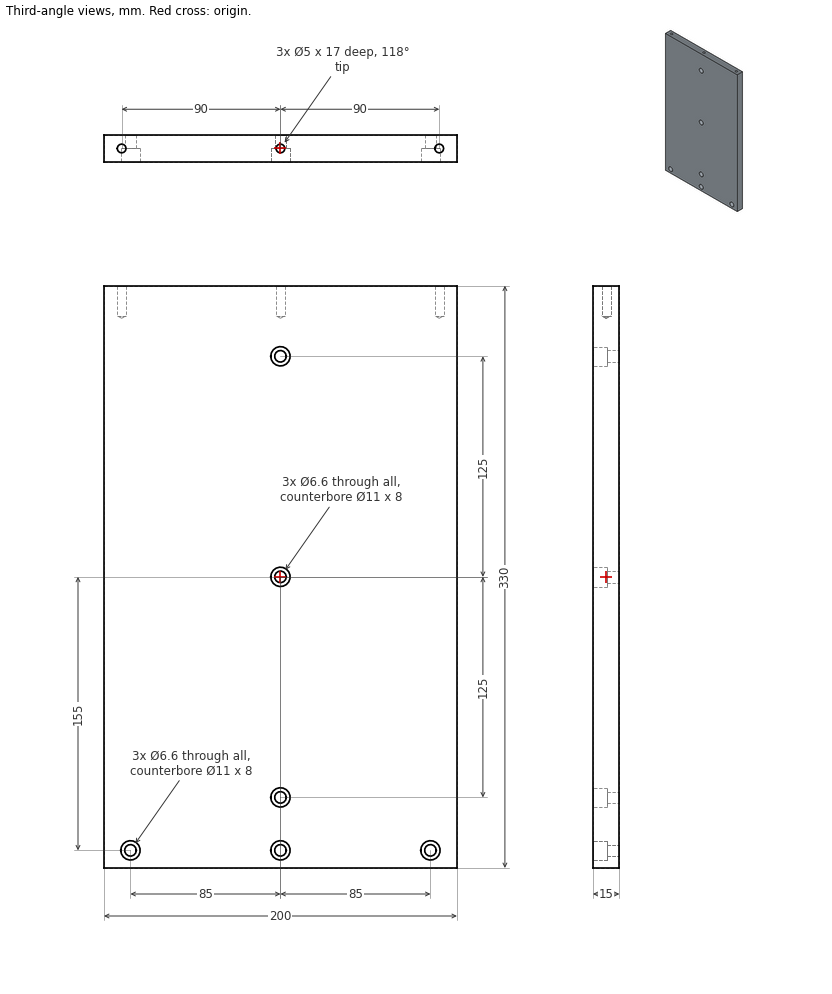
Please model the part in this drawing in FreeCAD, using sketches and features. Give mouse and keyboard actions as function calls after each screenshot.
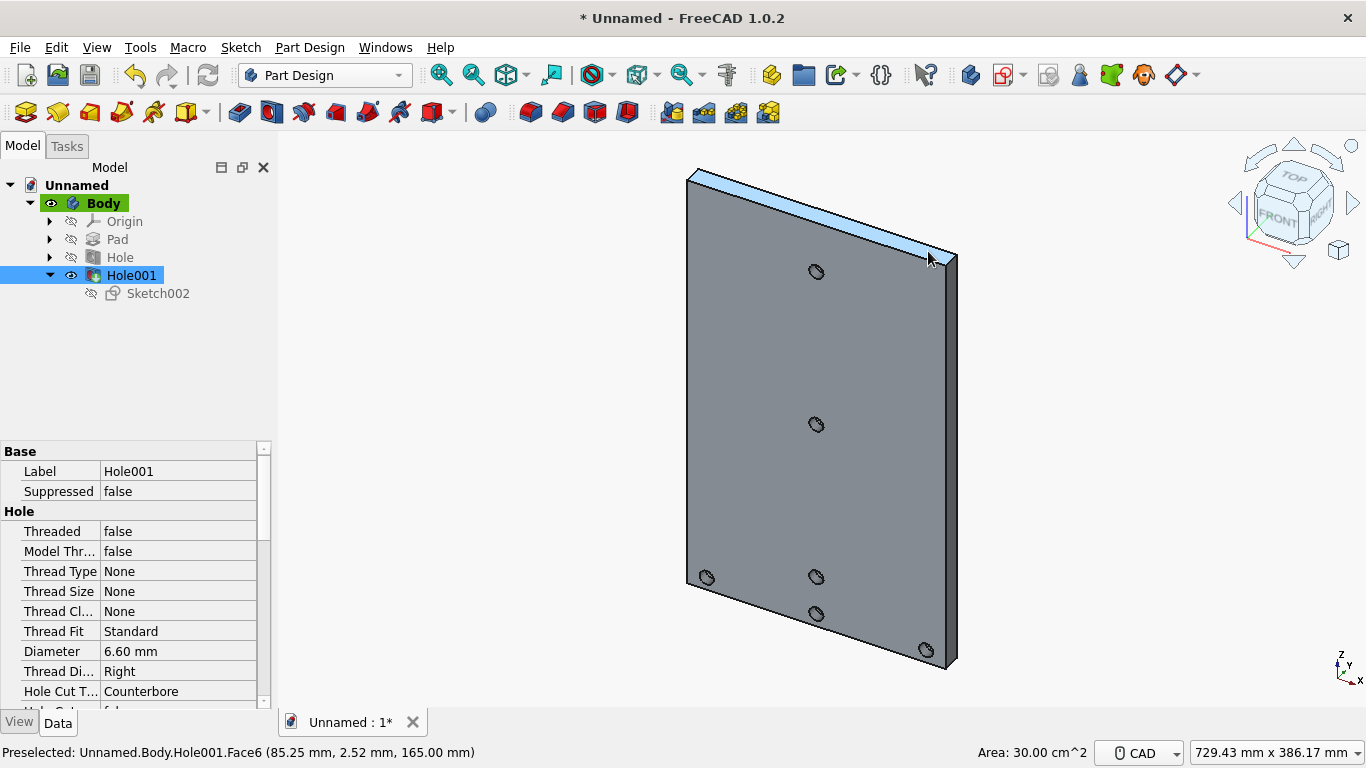
click(1004, 76)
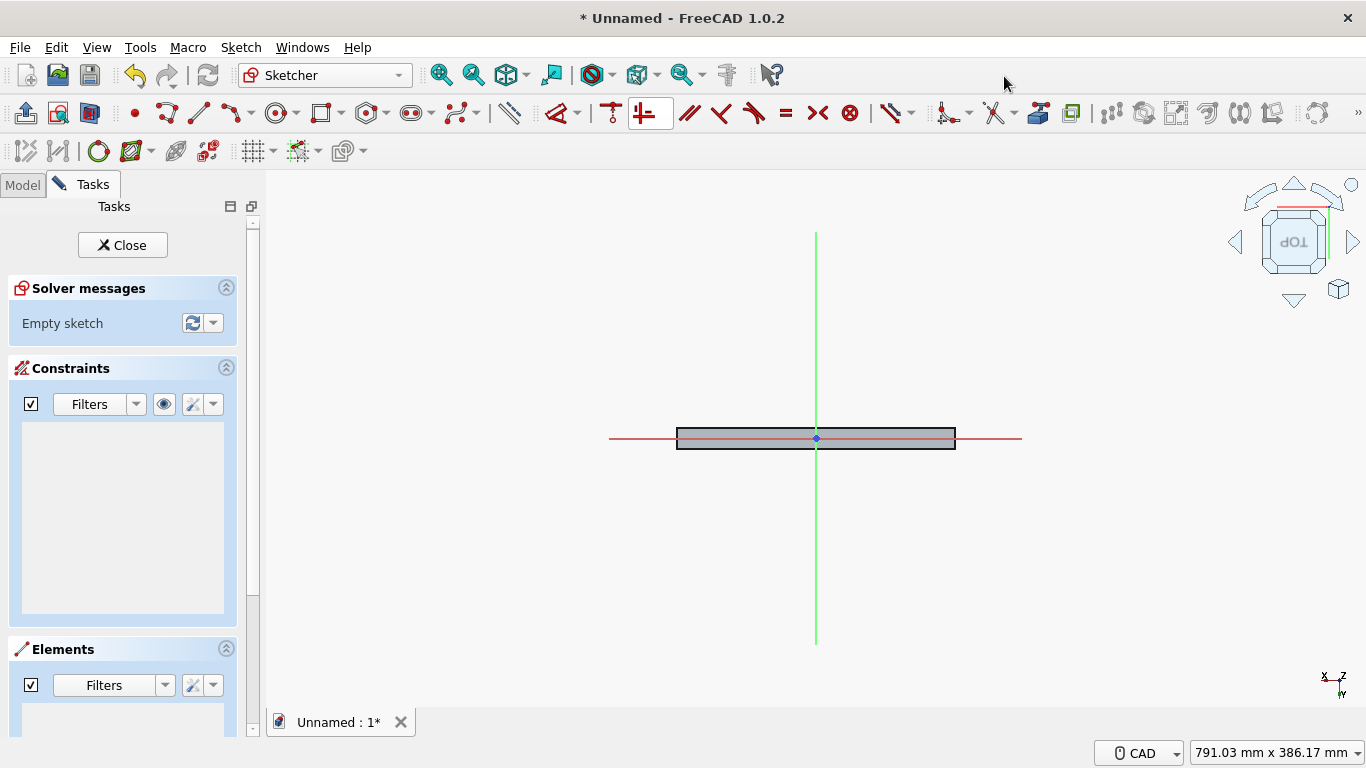
scroll(856, 439, up, 5)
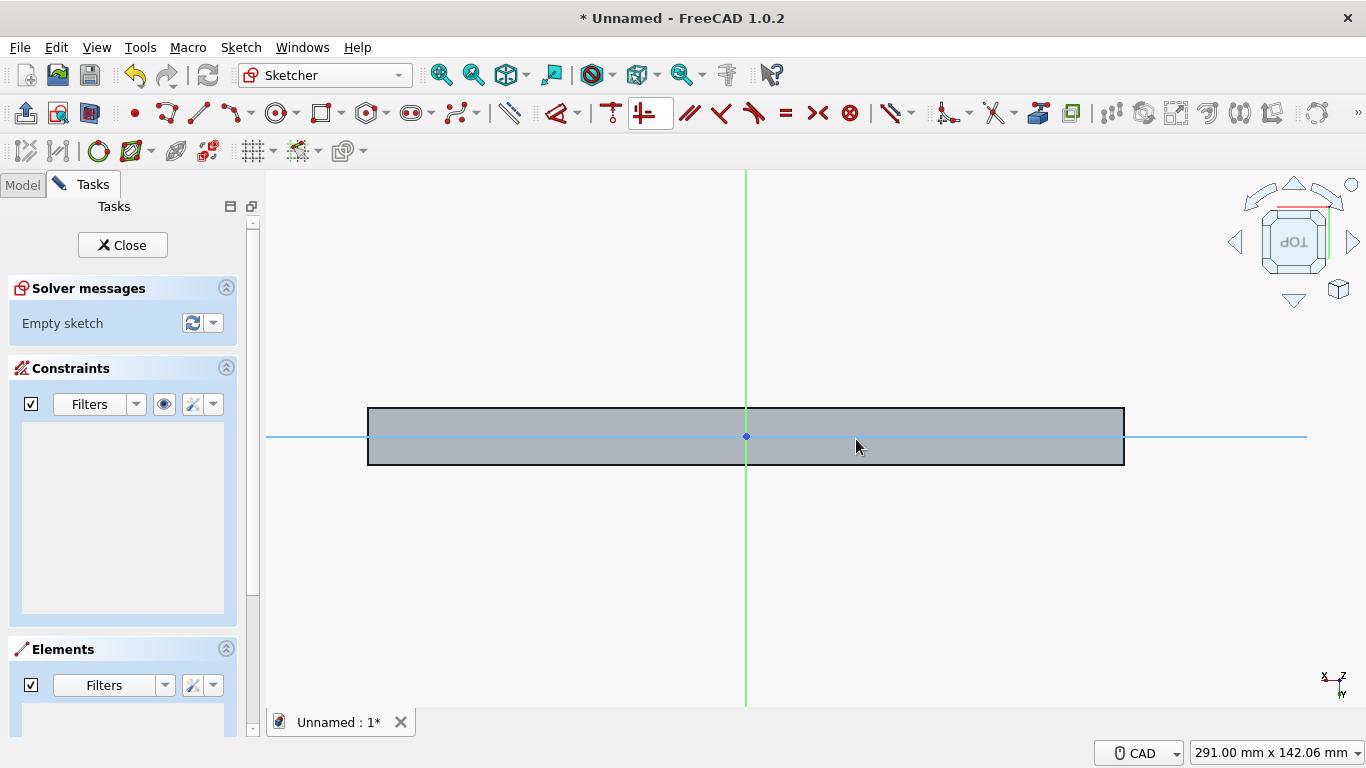
key(g)
key(c)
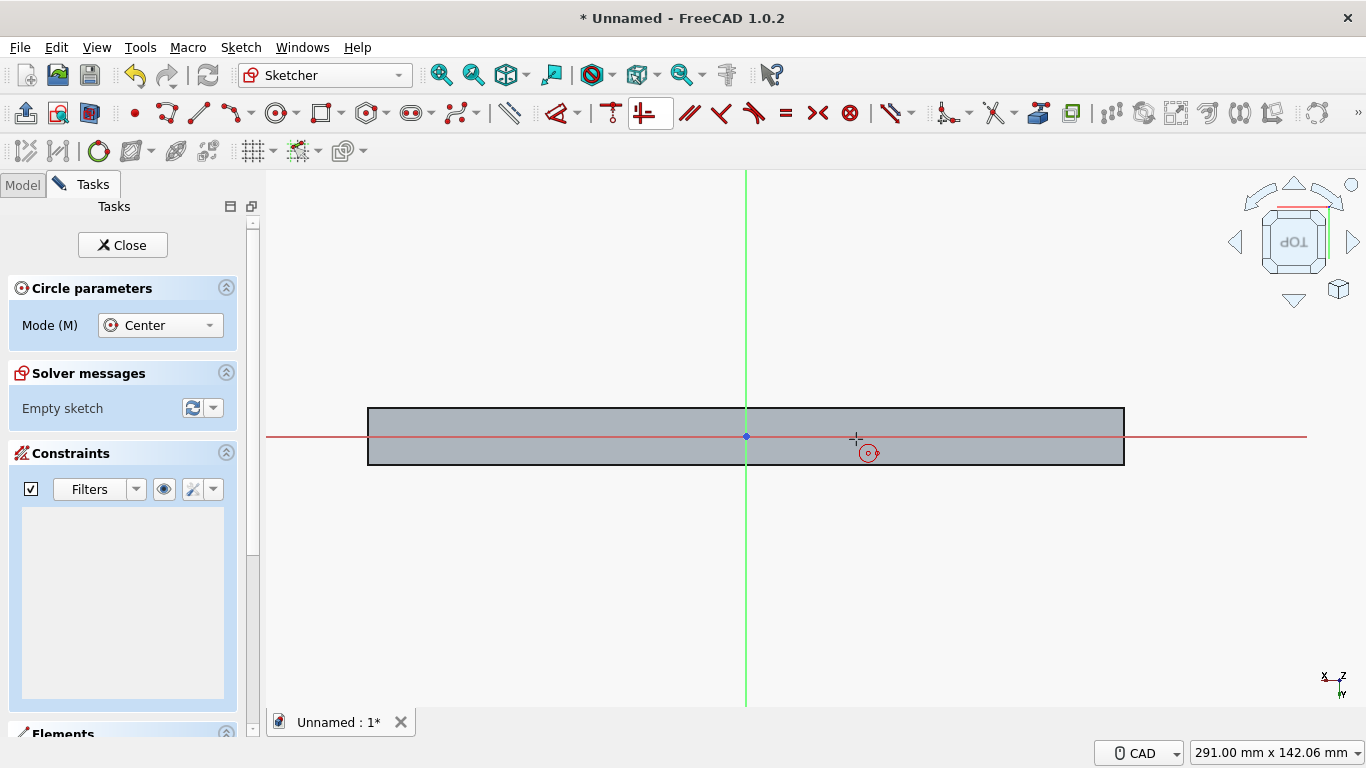
scroll(746, 437, up, 5)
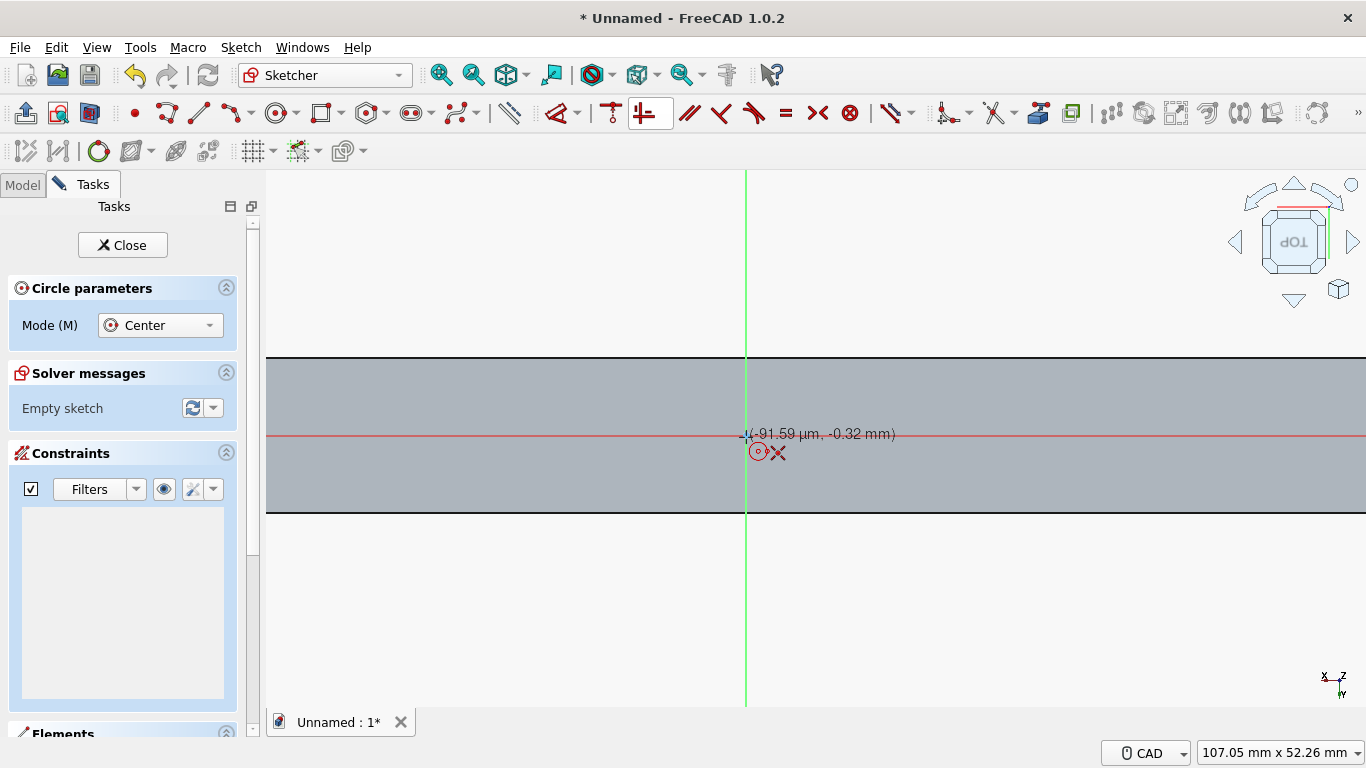
click(746, 436)
click(764, 417)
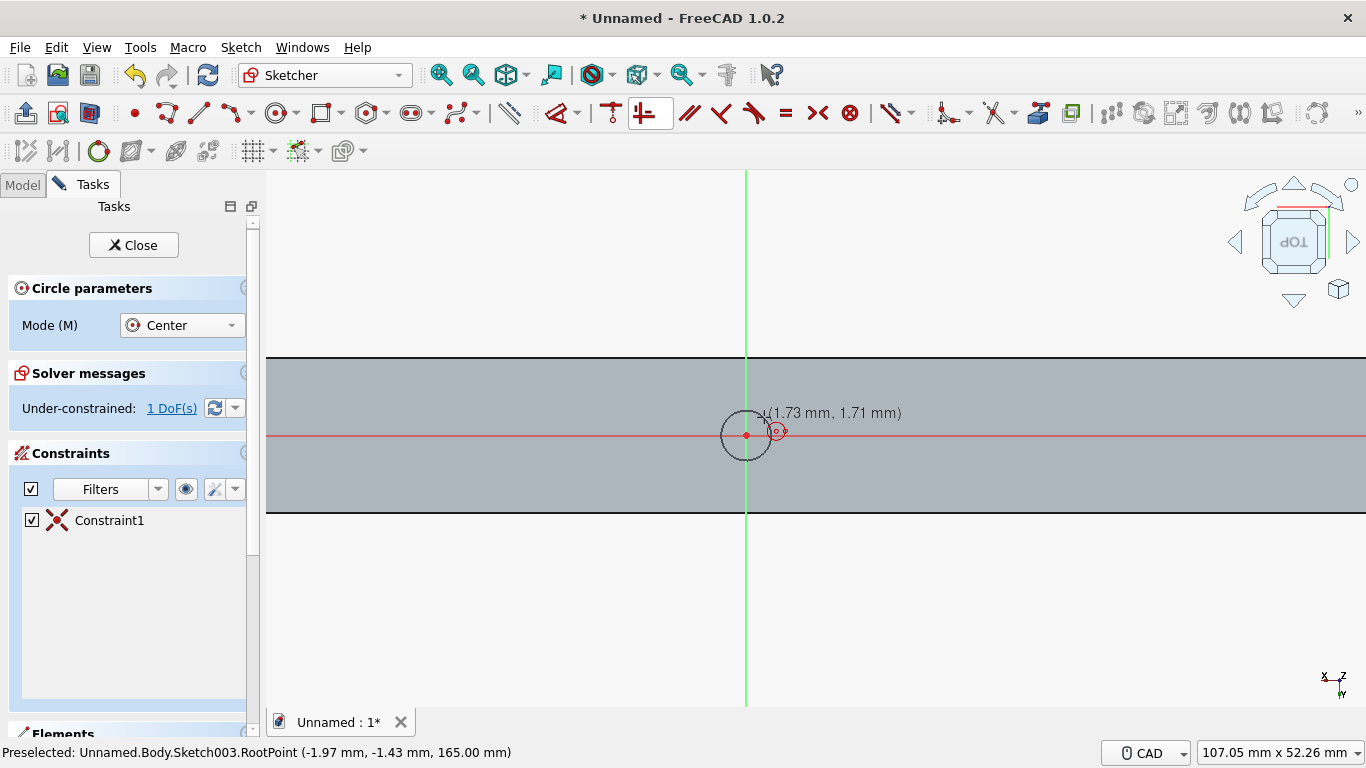
scroll(748, 440, down, 5)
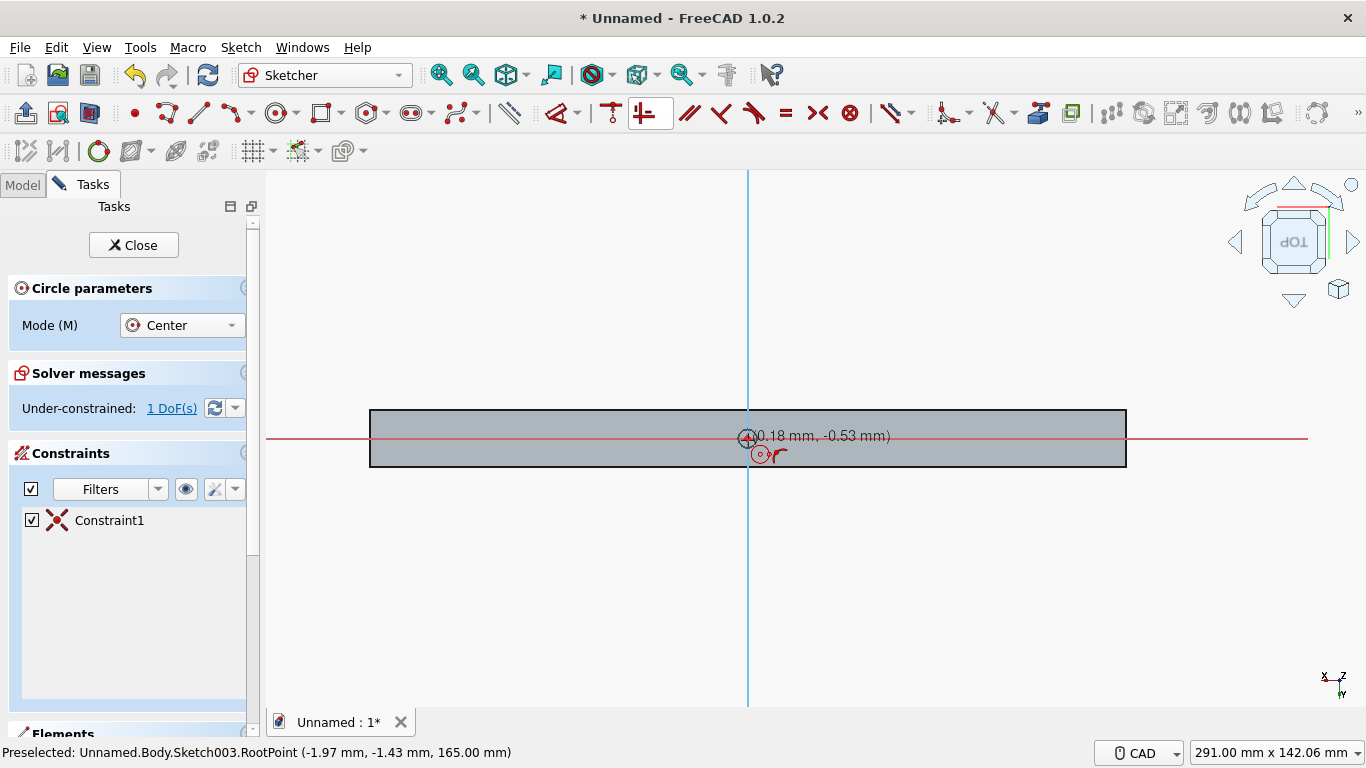
scroll(1088, 439, up, 5)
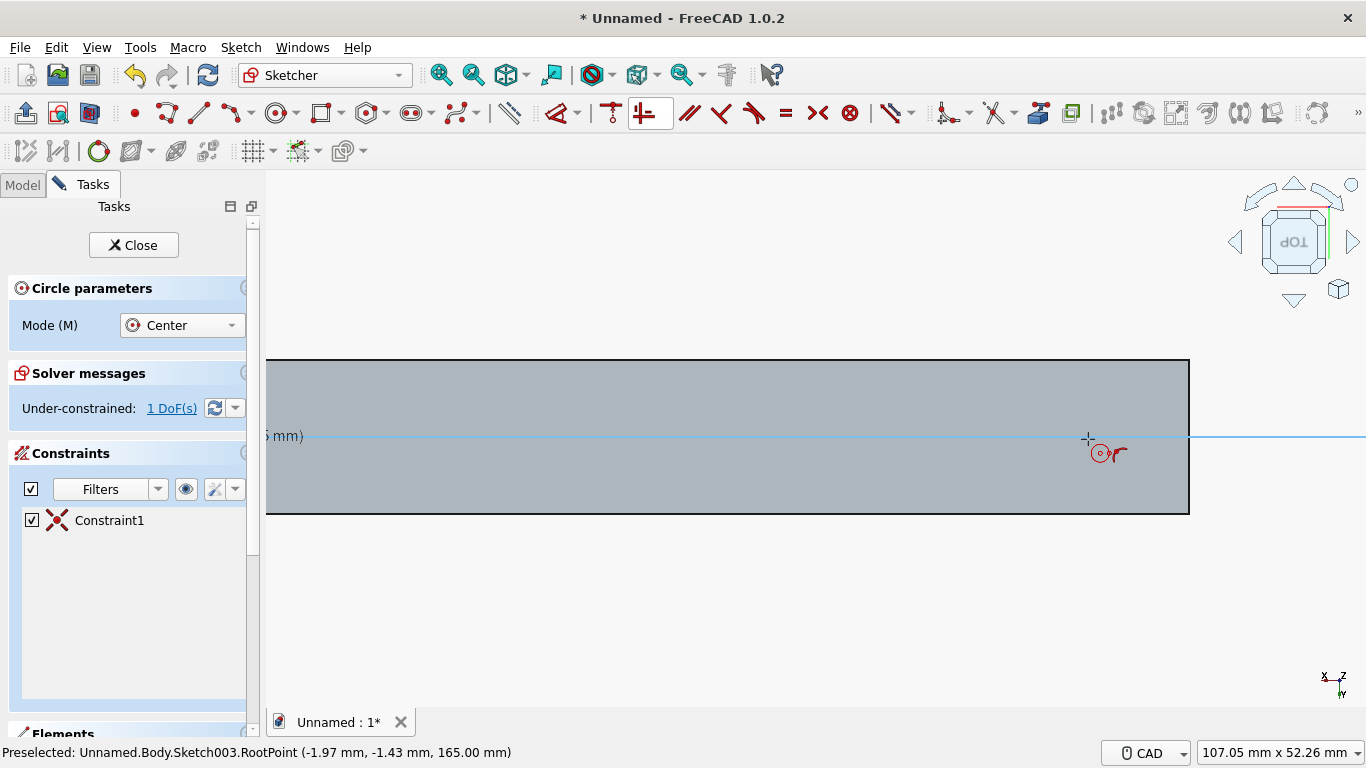
click(1086, 437)
click(1104, 419)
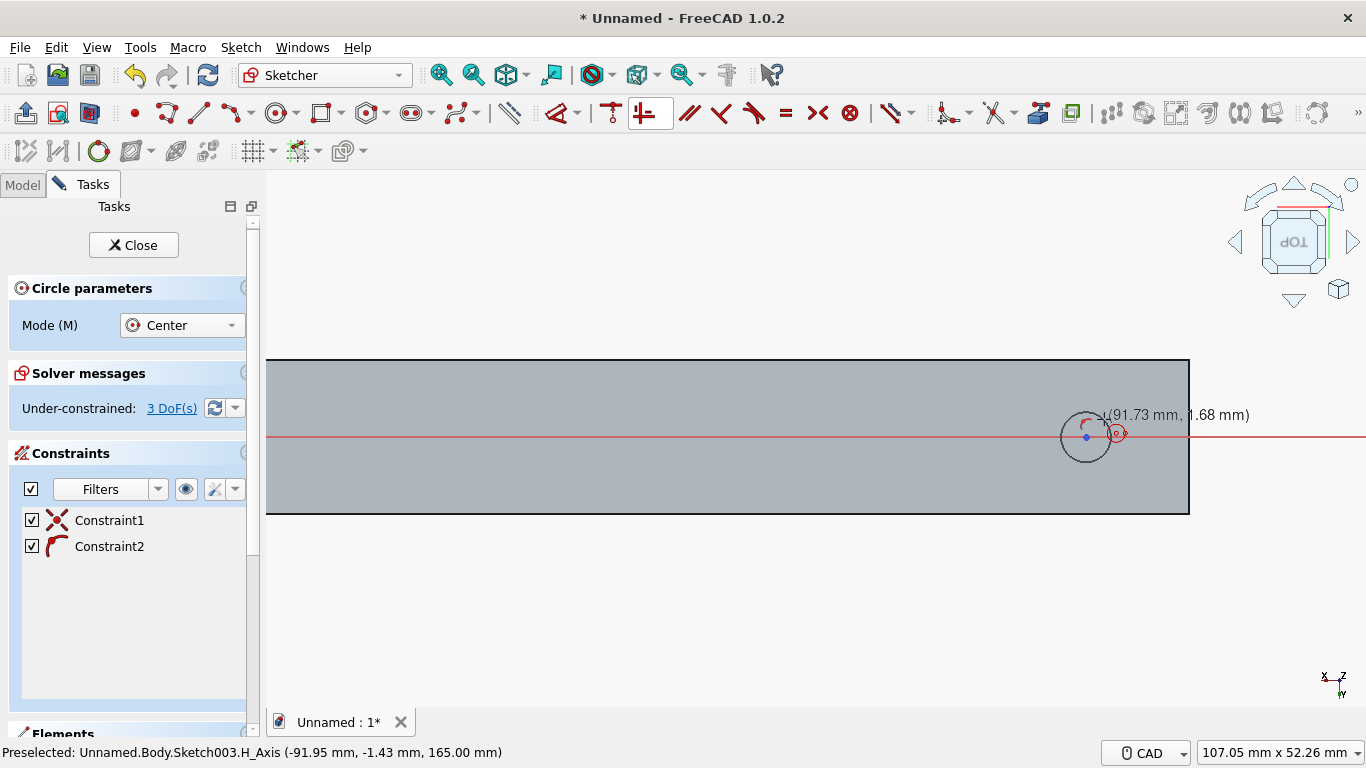
scroll(1089, 439, down, 5)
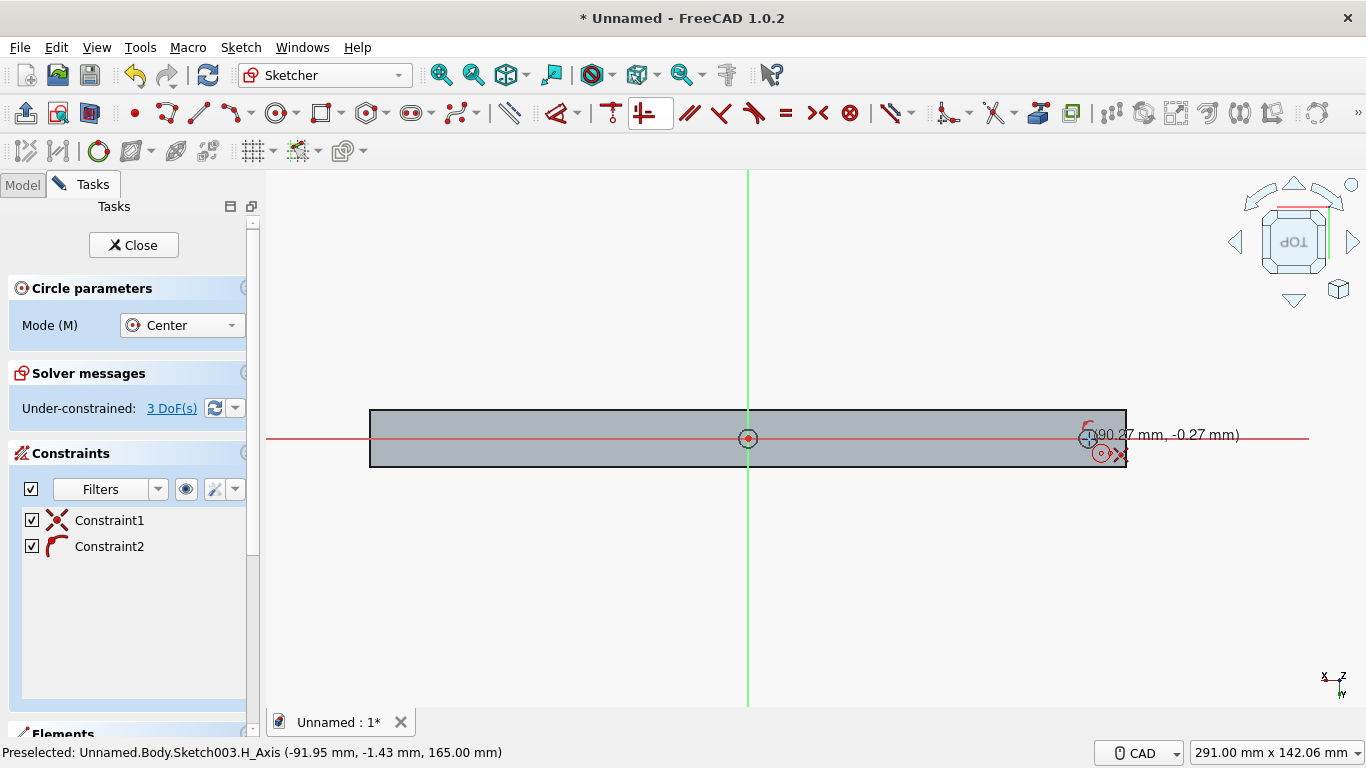
scroll(408, 439, up, 5)